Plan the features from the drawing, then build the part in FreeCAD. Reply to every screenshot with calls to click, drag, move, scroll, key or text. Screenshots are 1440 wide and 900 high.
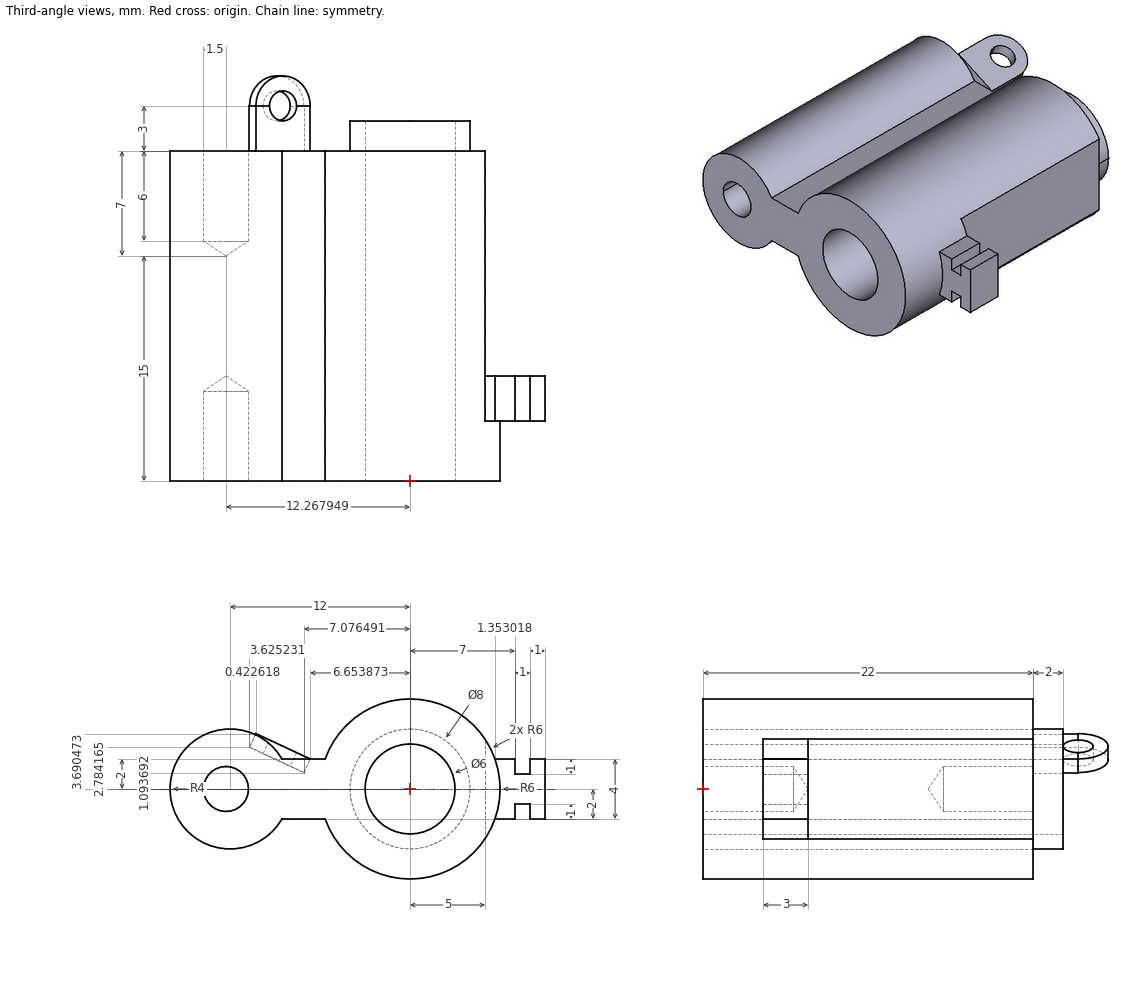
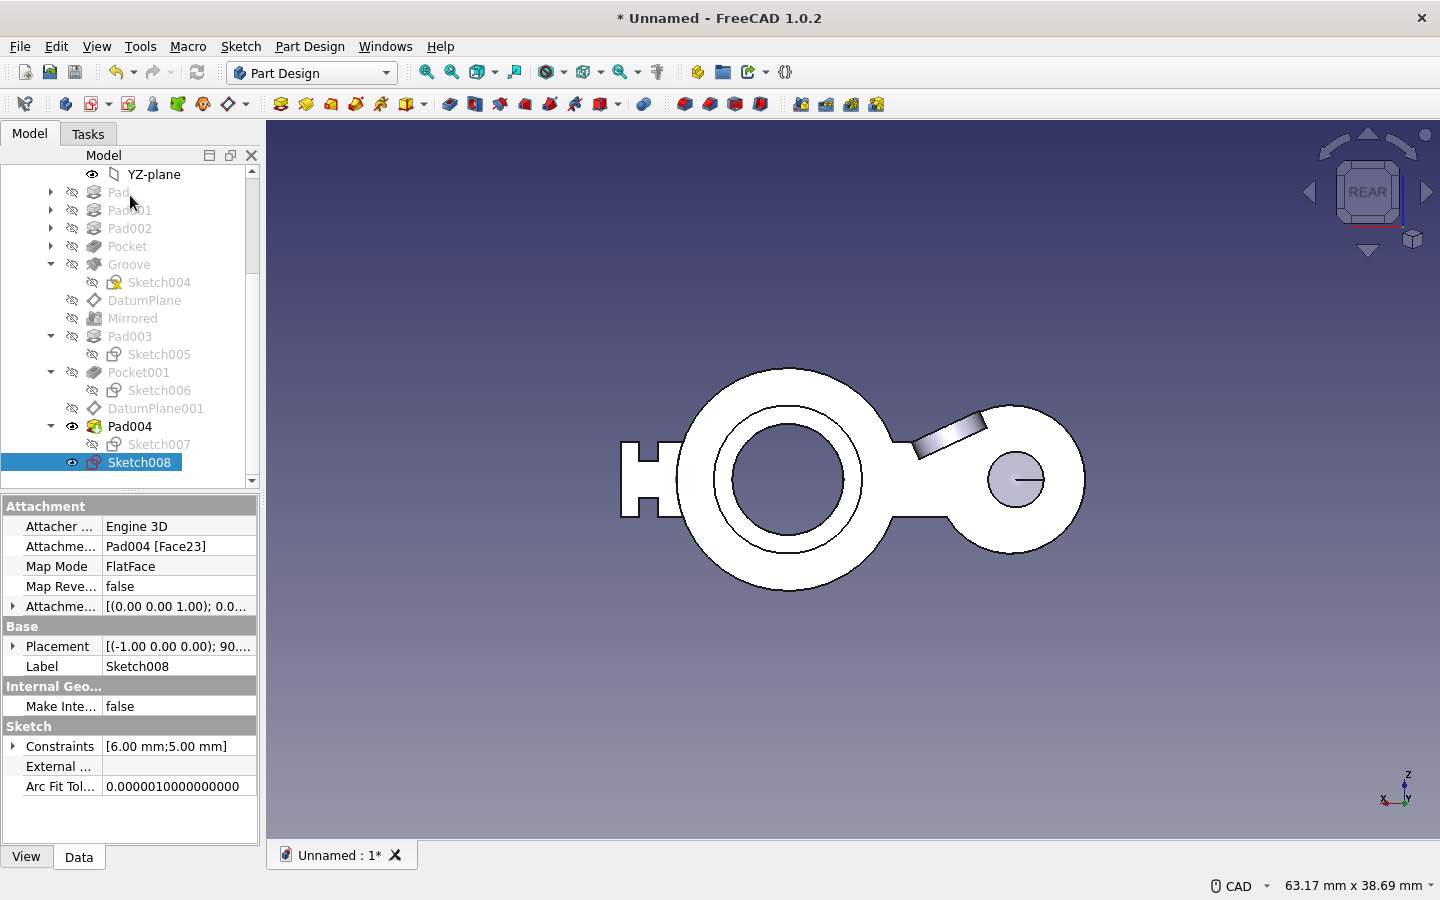
click(450, 104)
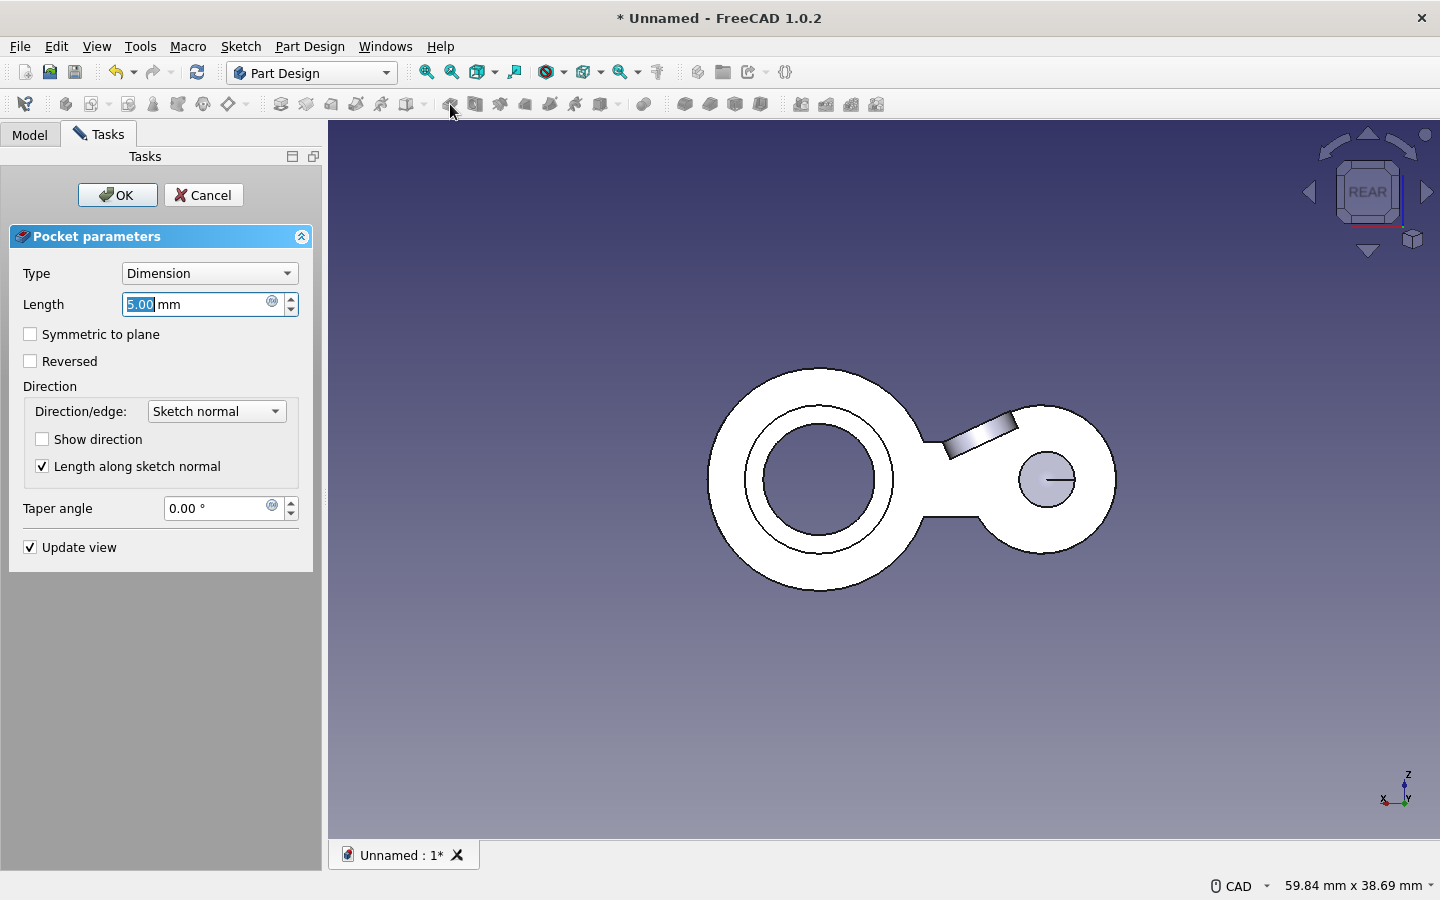
click(210, 274)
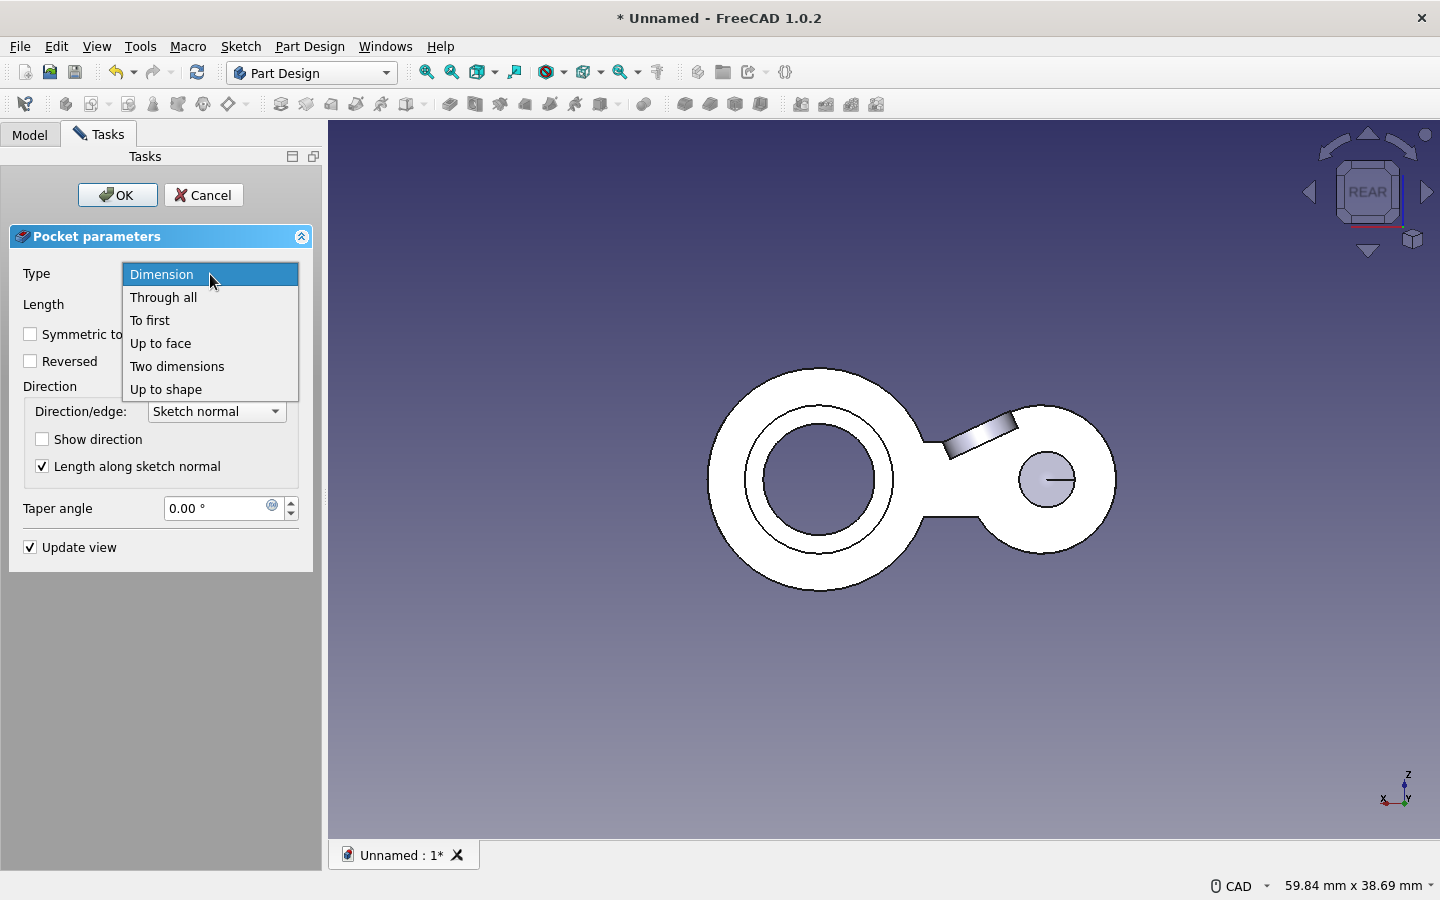
click(208, 298)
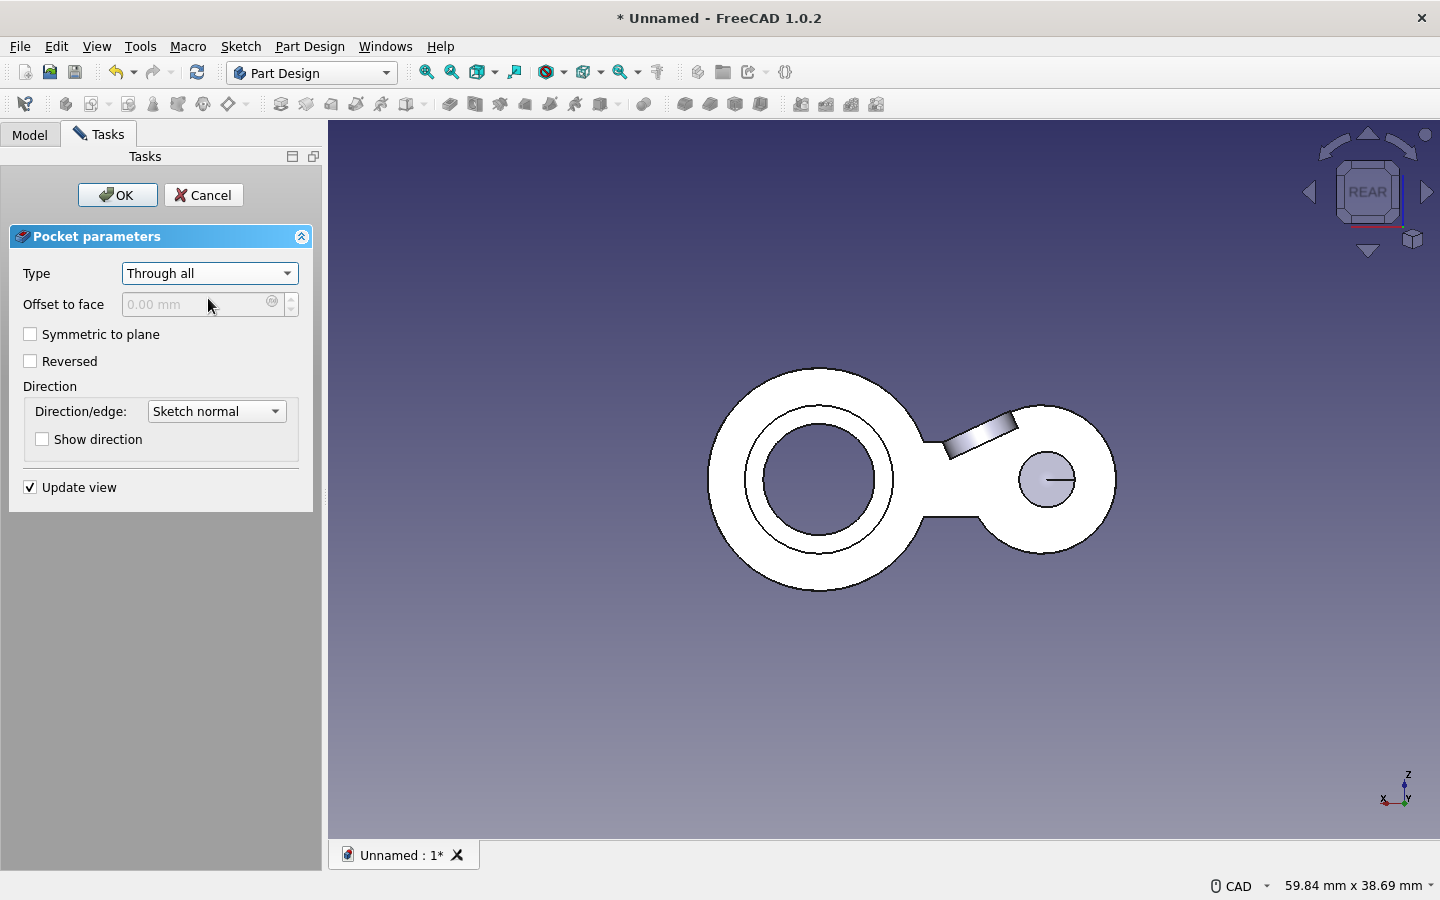
click(31, 361)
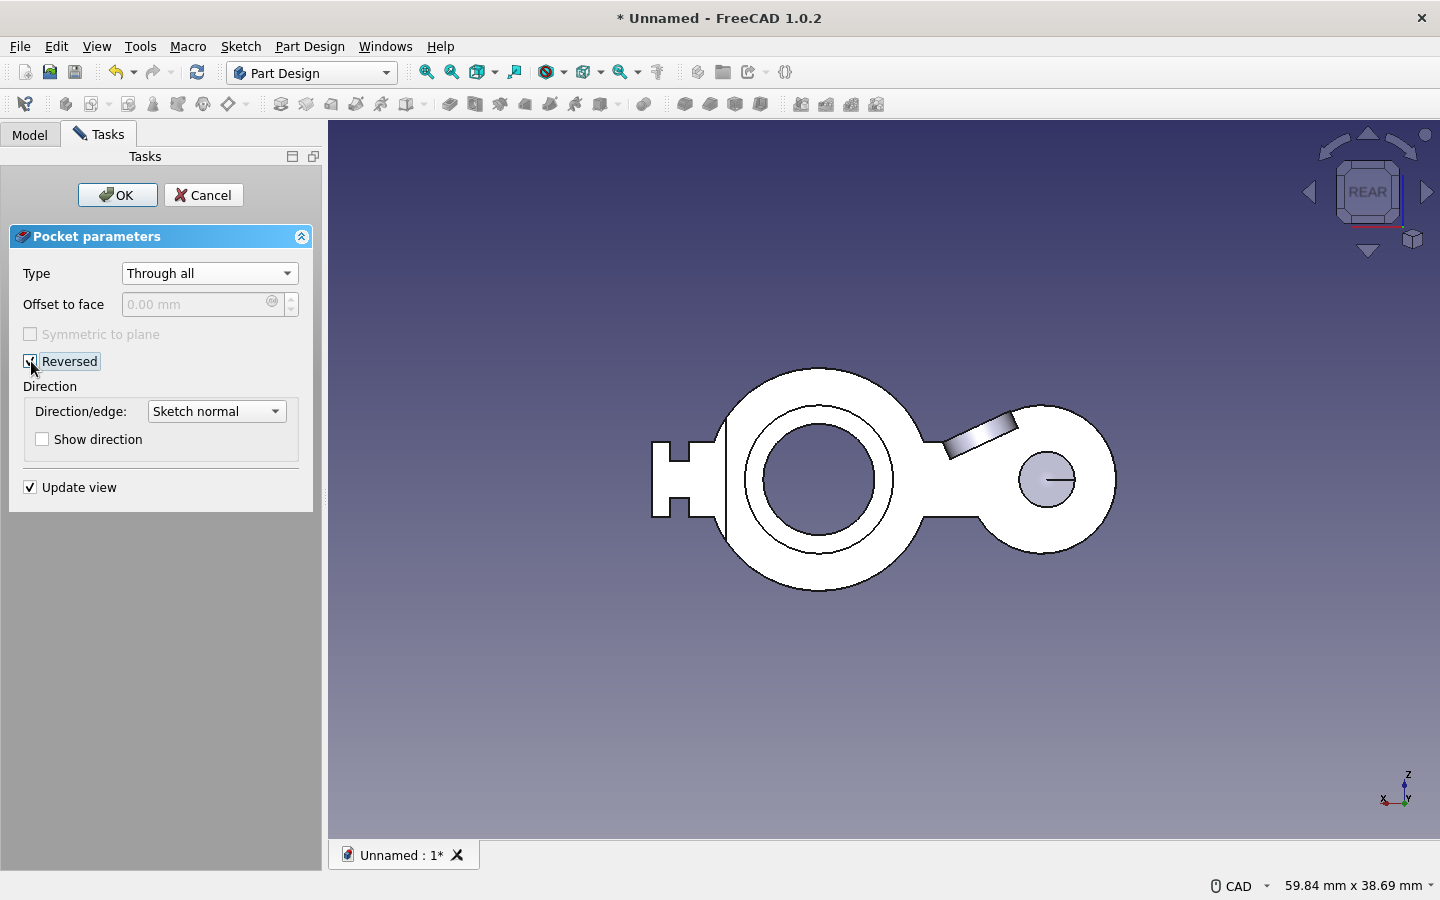
click(118, 195)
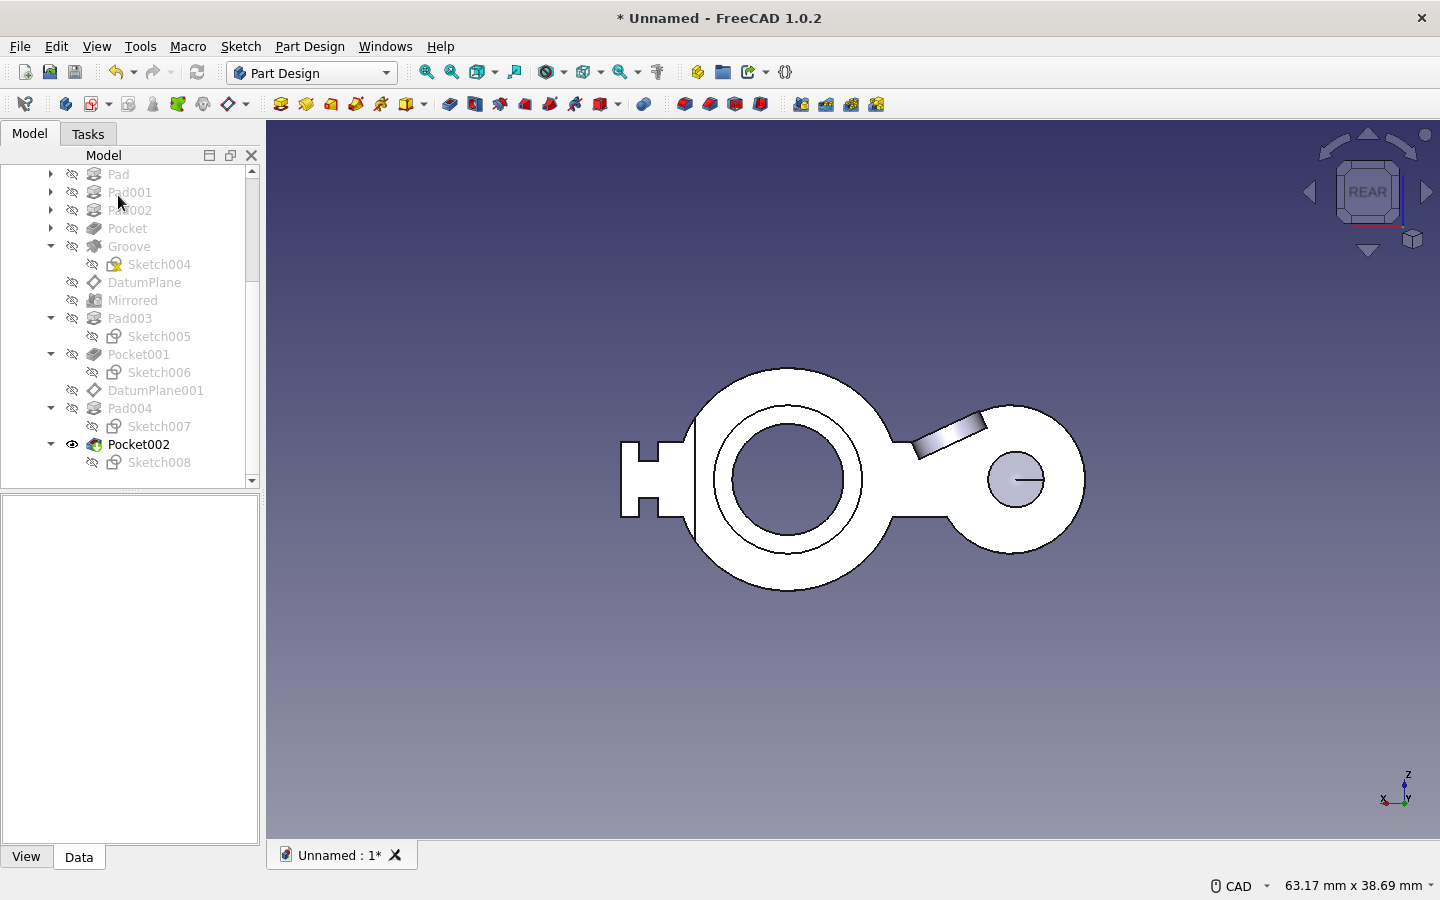
key(0)